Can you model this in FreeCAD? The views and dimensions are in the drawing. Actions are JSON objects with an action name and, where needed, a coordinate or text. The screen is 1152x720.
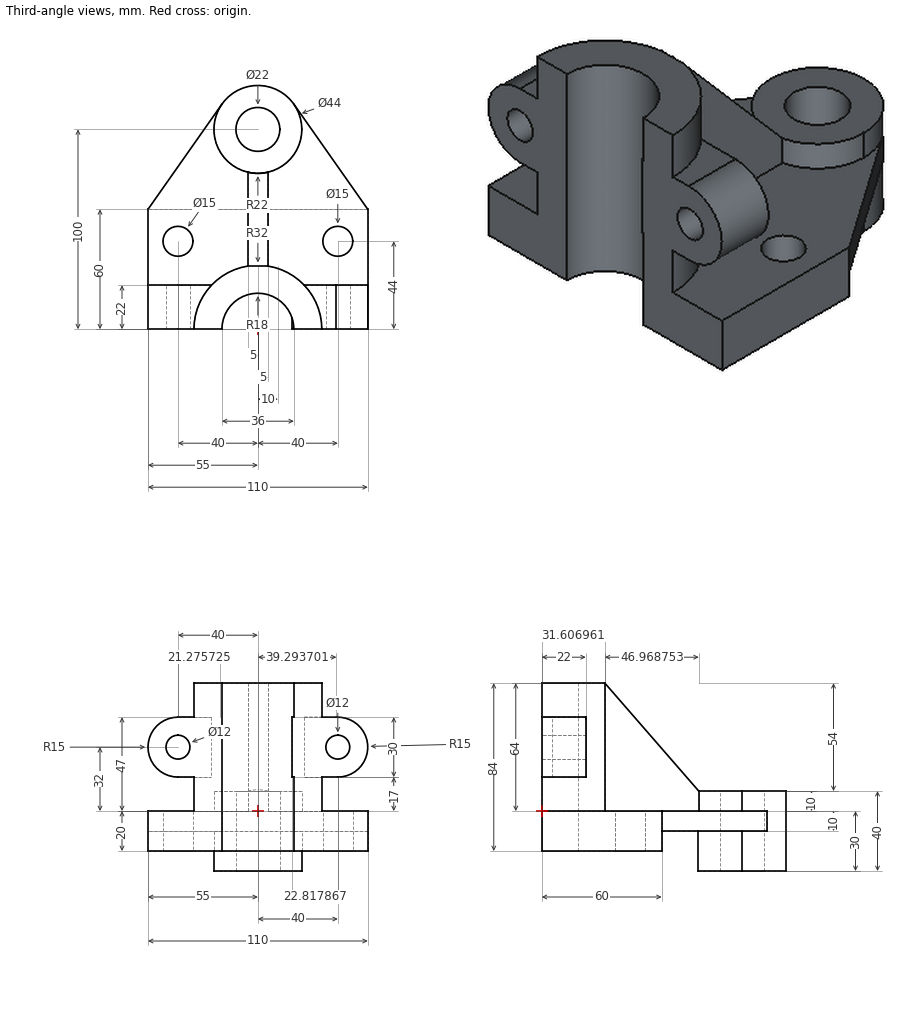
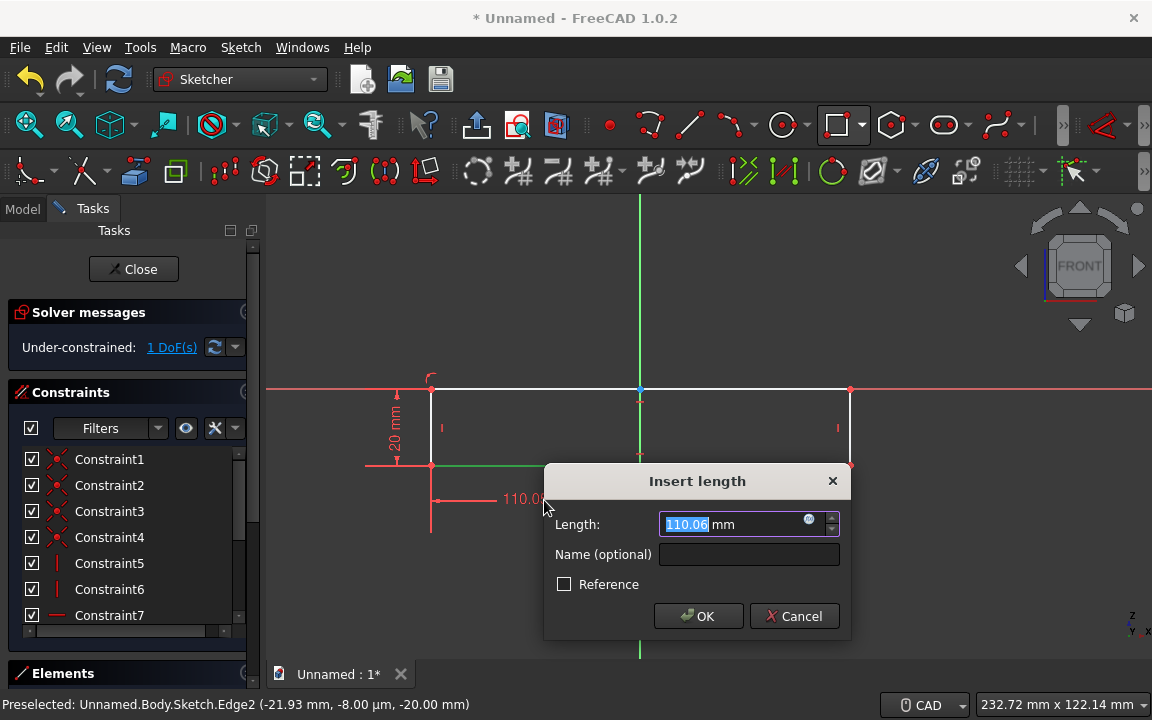
{"action": "type", "text": "110"}
{"action": "key", "text": "Return"}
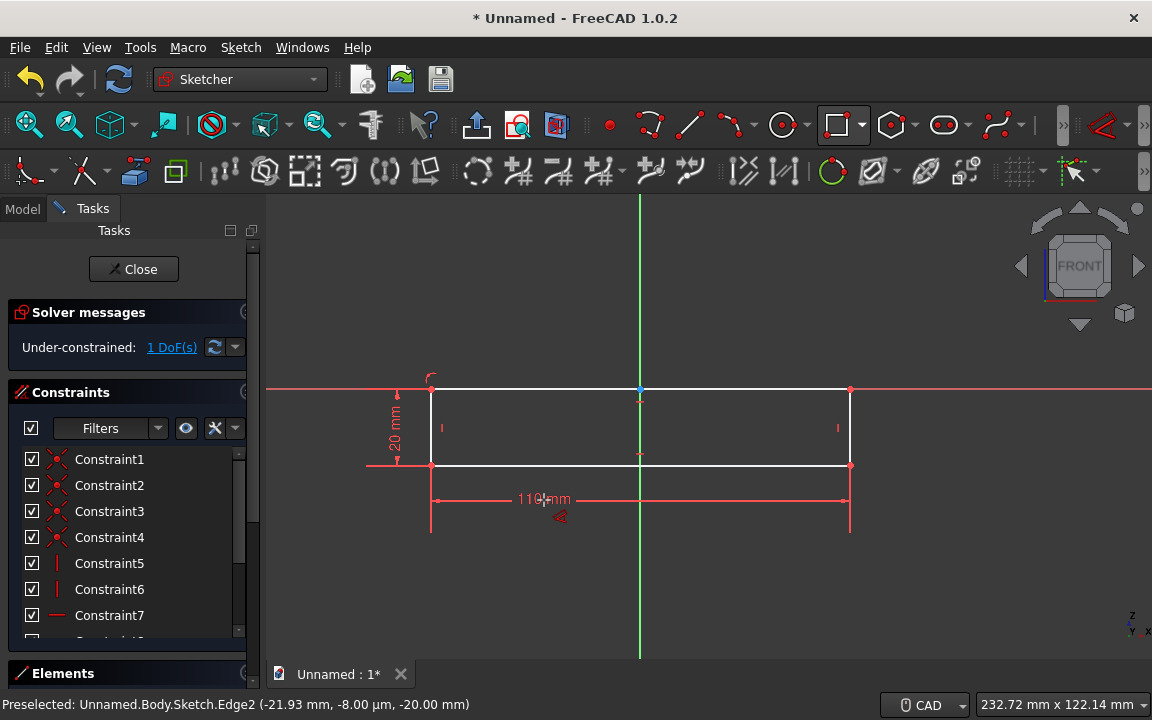
{"action": "left_click", "coordinate": [431, 389]}
{"action": "left_click", "coordinate": [536, 355]}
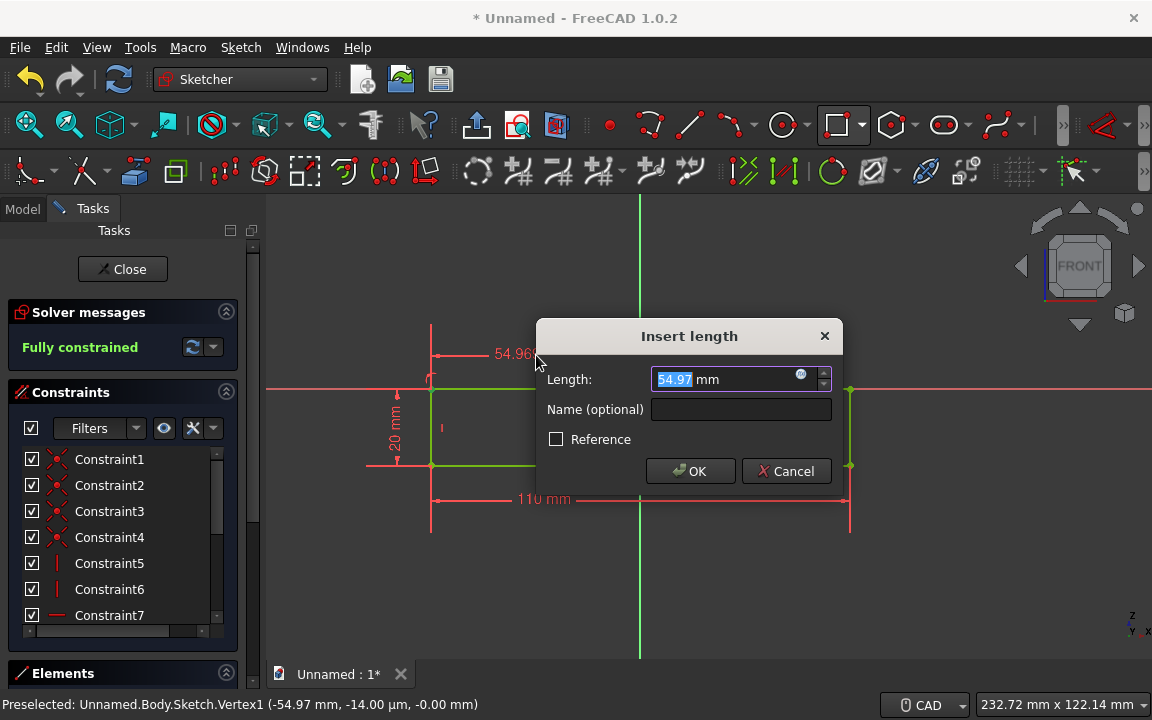
{"action": "type", "text": "55"}
{"action": "key", "text": "Return"}
{"action": "key", "text": "Escape"}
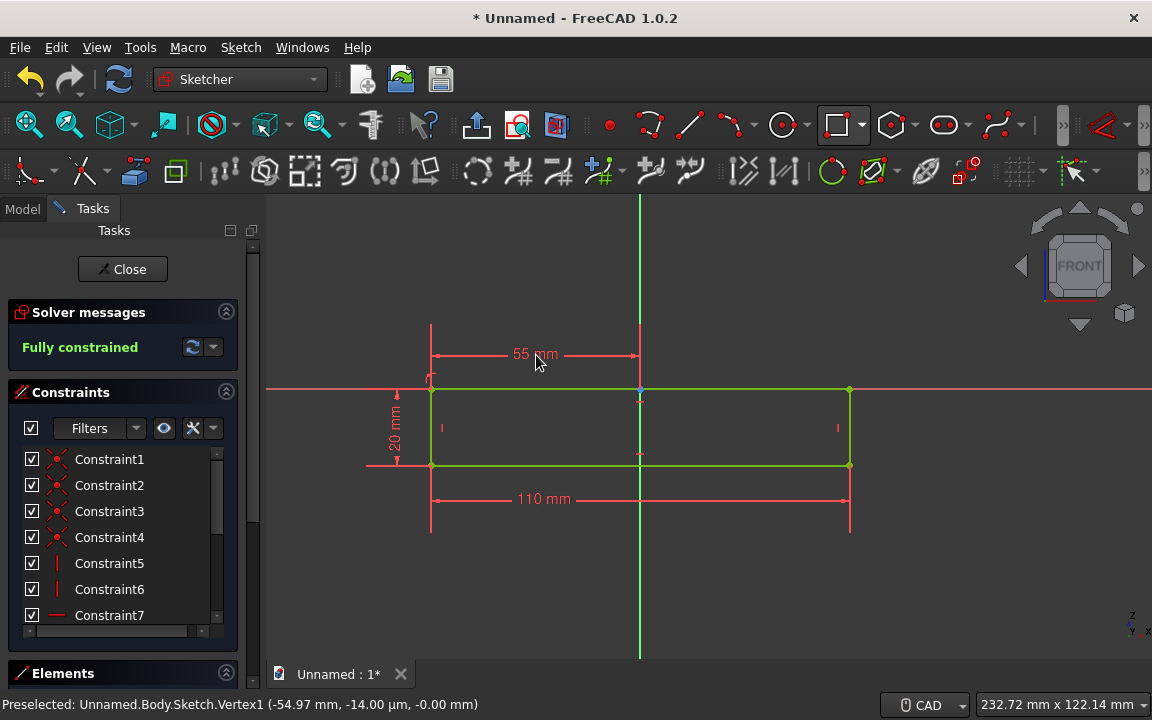
{"action": "left_click", "coordinate": [123, 269]}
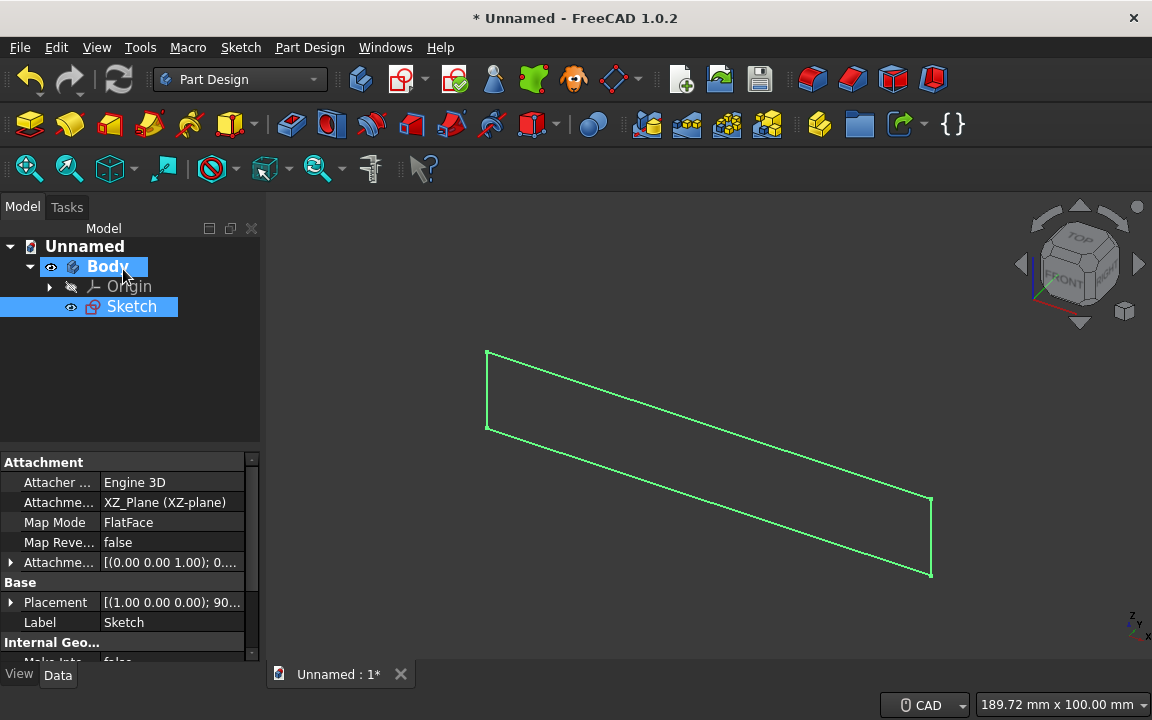
{"action": "left_click", "coordinate": [30, 124]}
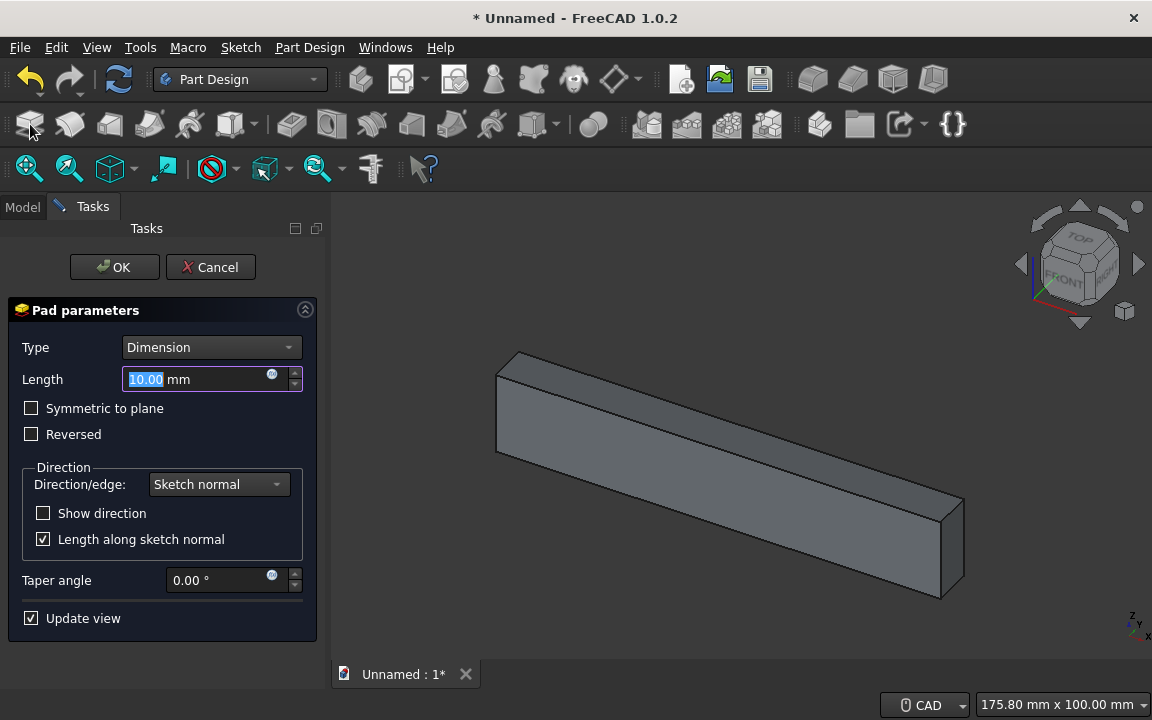
{"action": "type", "text": "60"}
{"action": "key", "text": "Tab"}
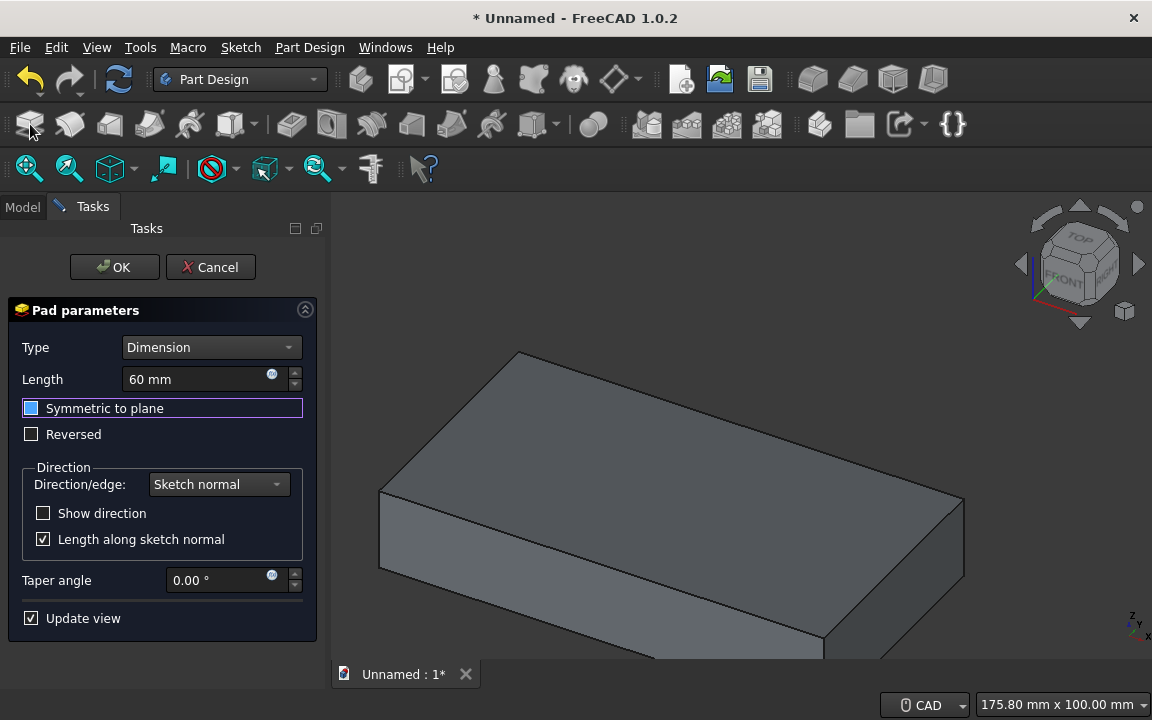
{"action": "left_click", "coordinate": [30, 434]}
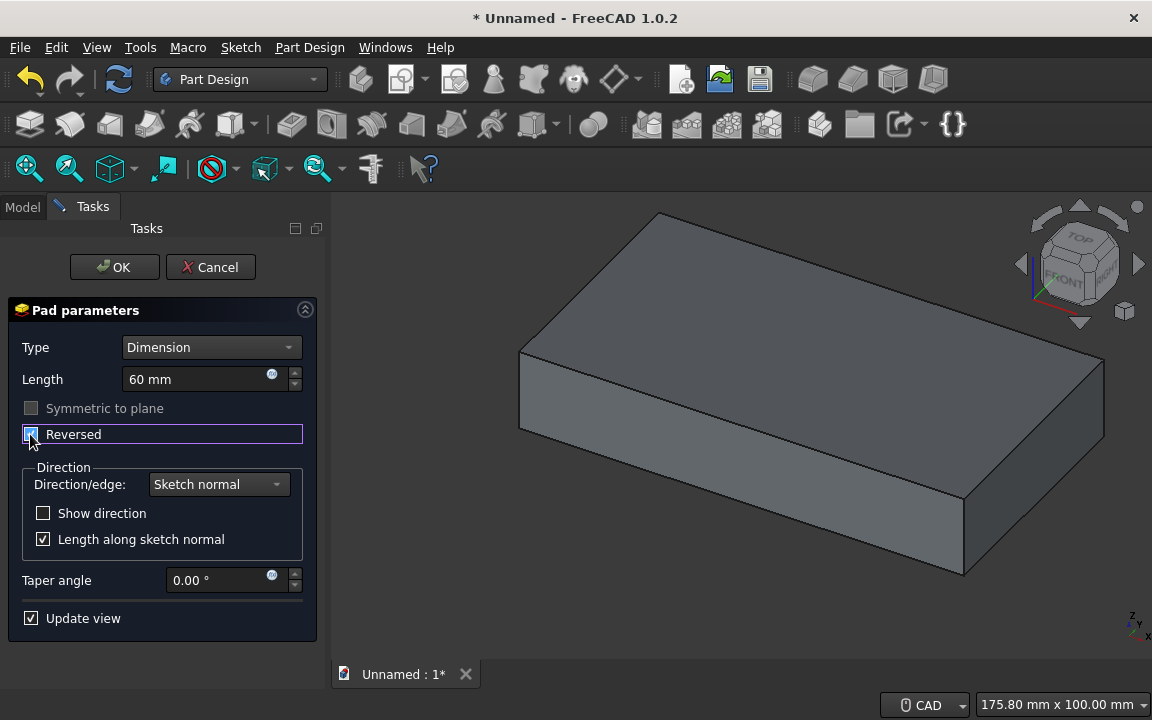
{"action": "left_click", "coordinate": [115, 267]}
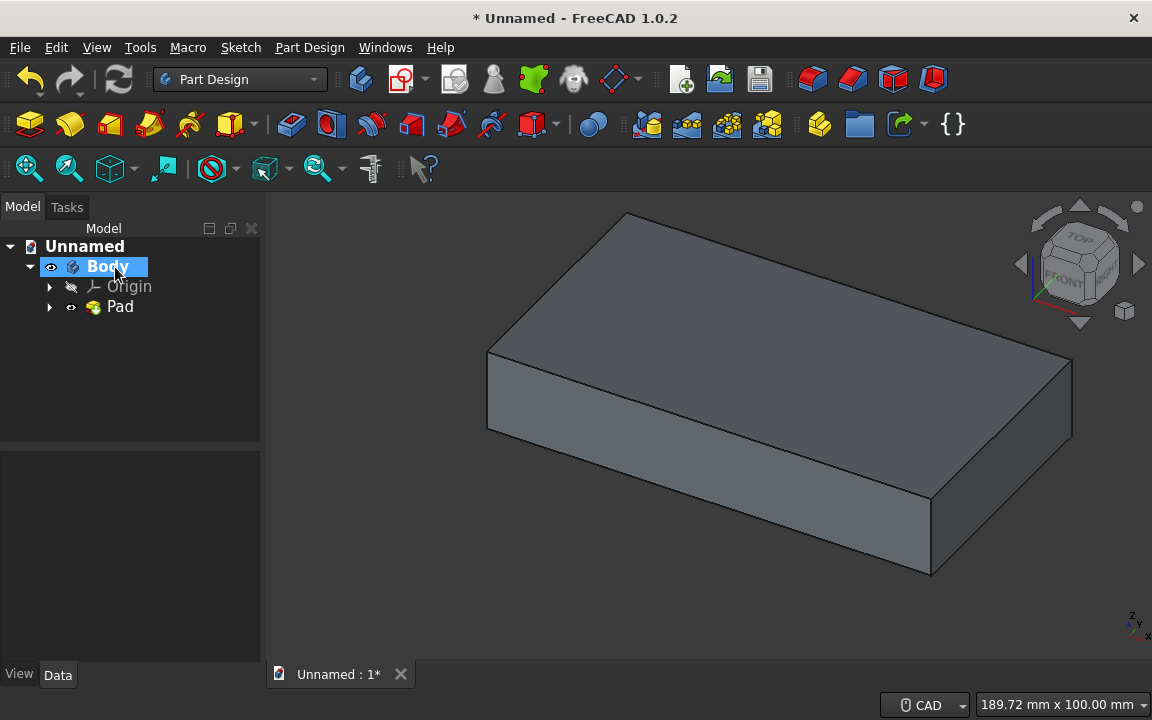
{"action": "left_click", "coordinate": [843, 376]}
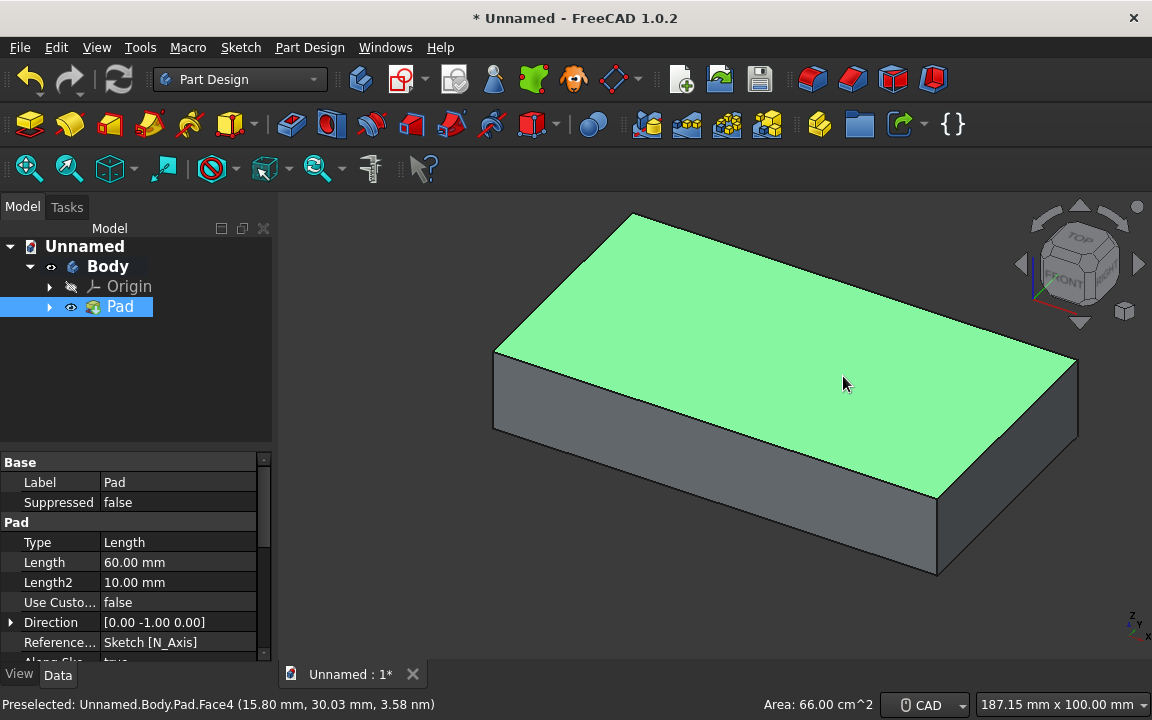
{"action": "left_click", "coordinate": [402, 80]}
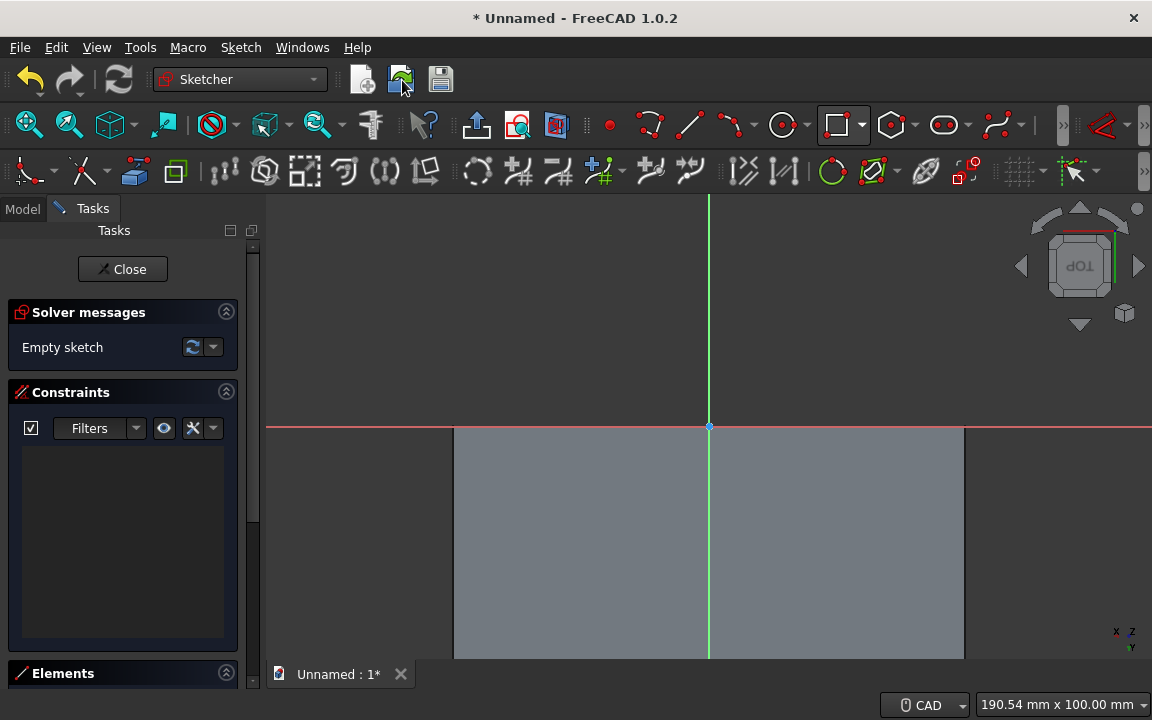
{"action": "scroll", "coordinate": [848, 631], "scroll_direction": "up", "scroll_amount": 2}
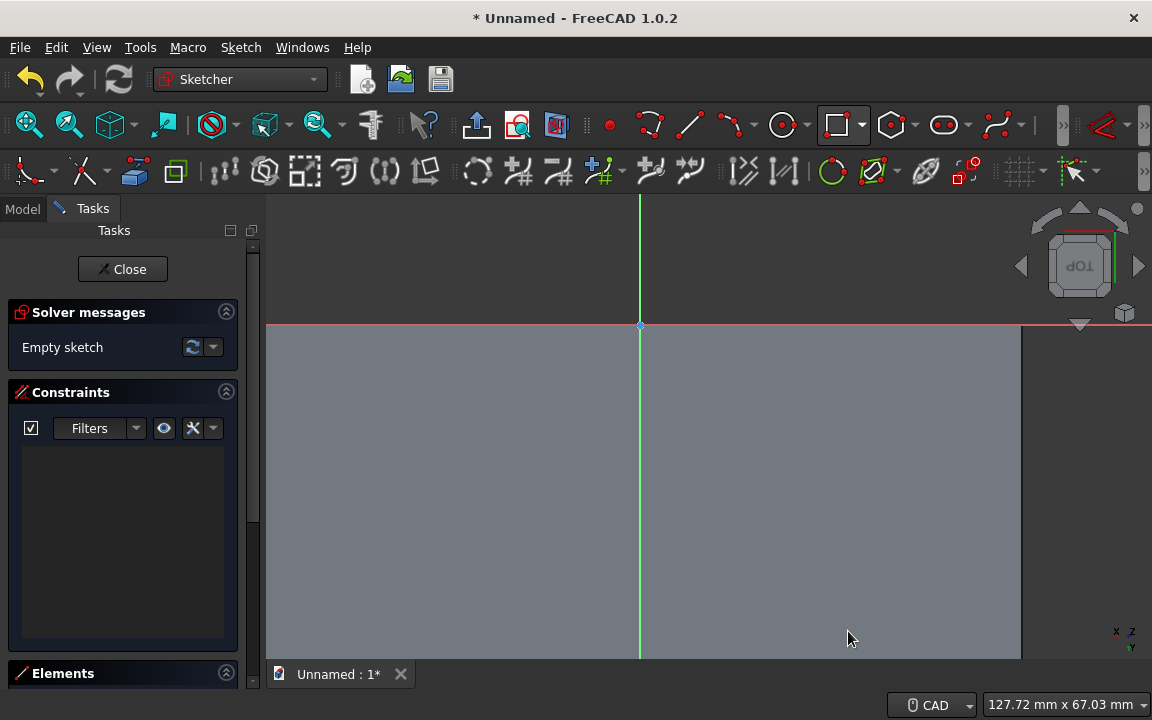
{"action": "left_click", "coordinate": [690, 126]}